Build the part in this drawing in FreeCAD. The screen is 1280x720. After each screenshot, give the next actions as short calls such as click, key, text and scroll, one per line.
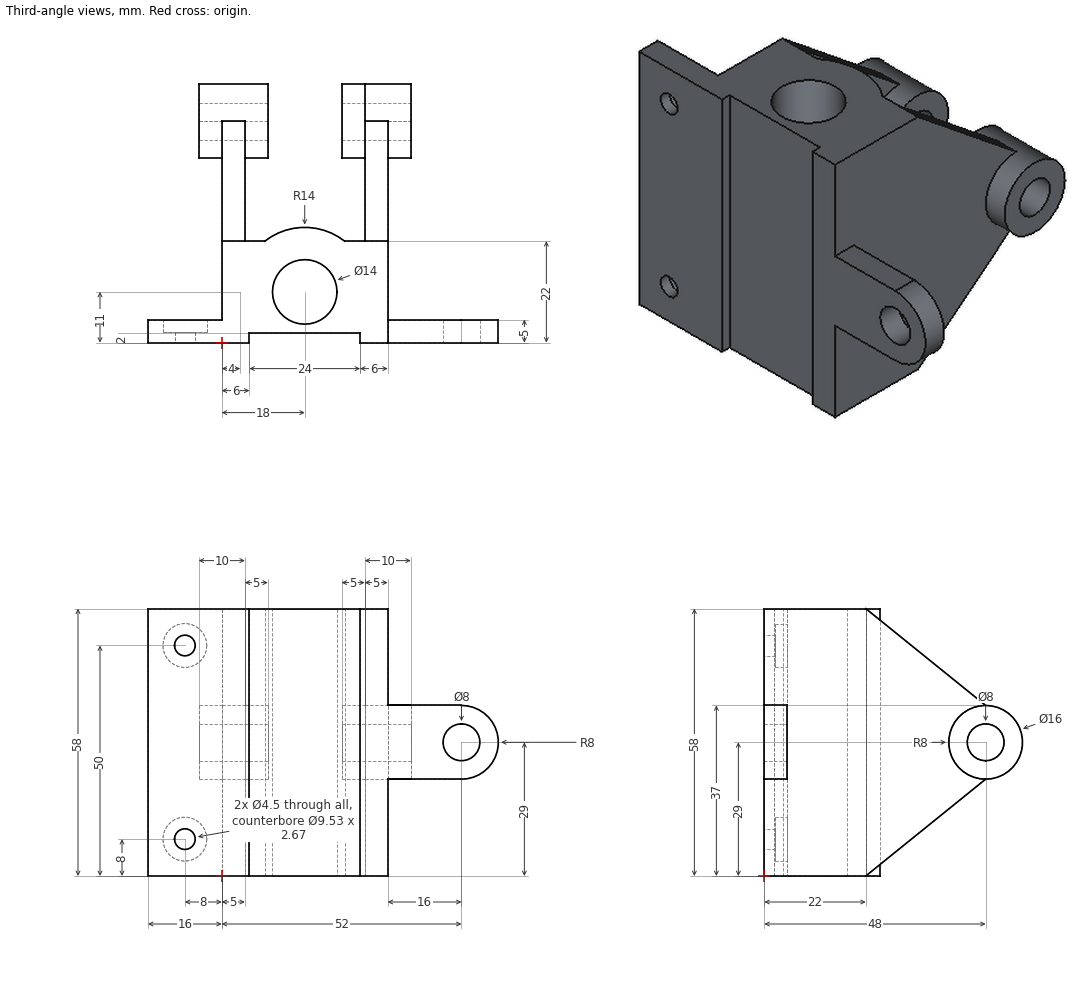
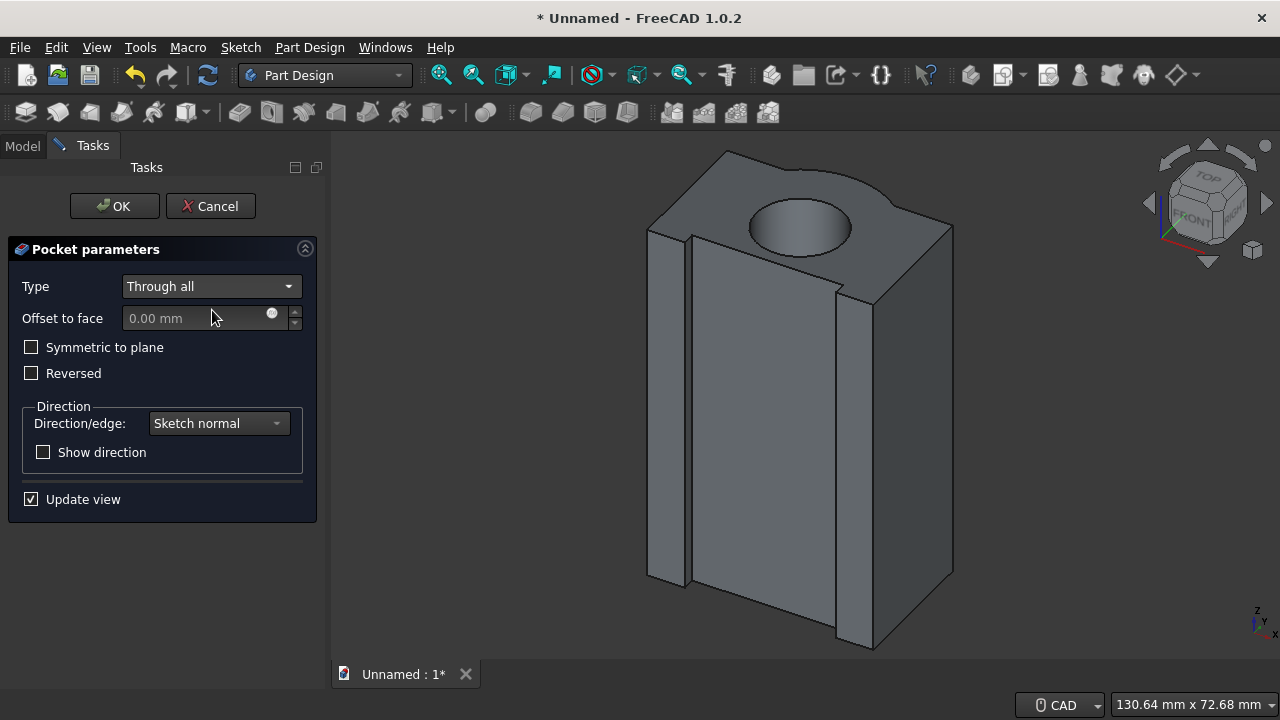
click(115, 206)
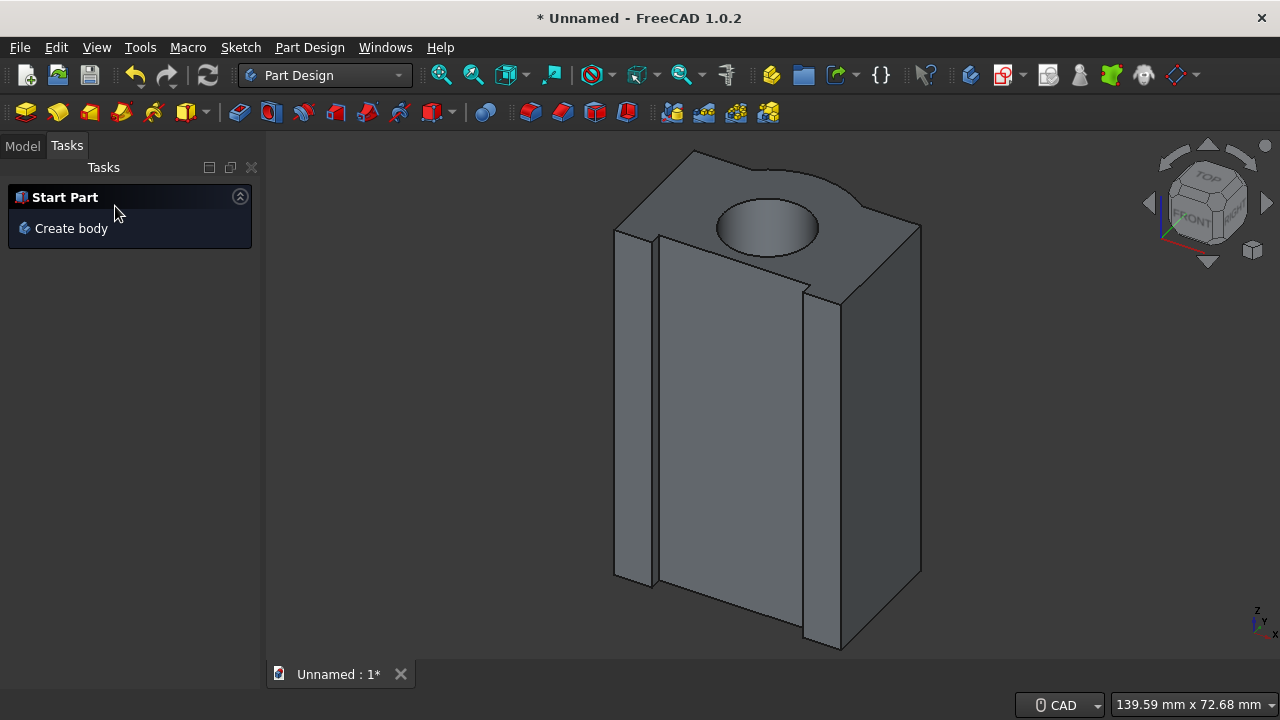
click(972, 76)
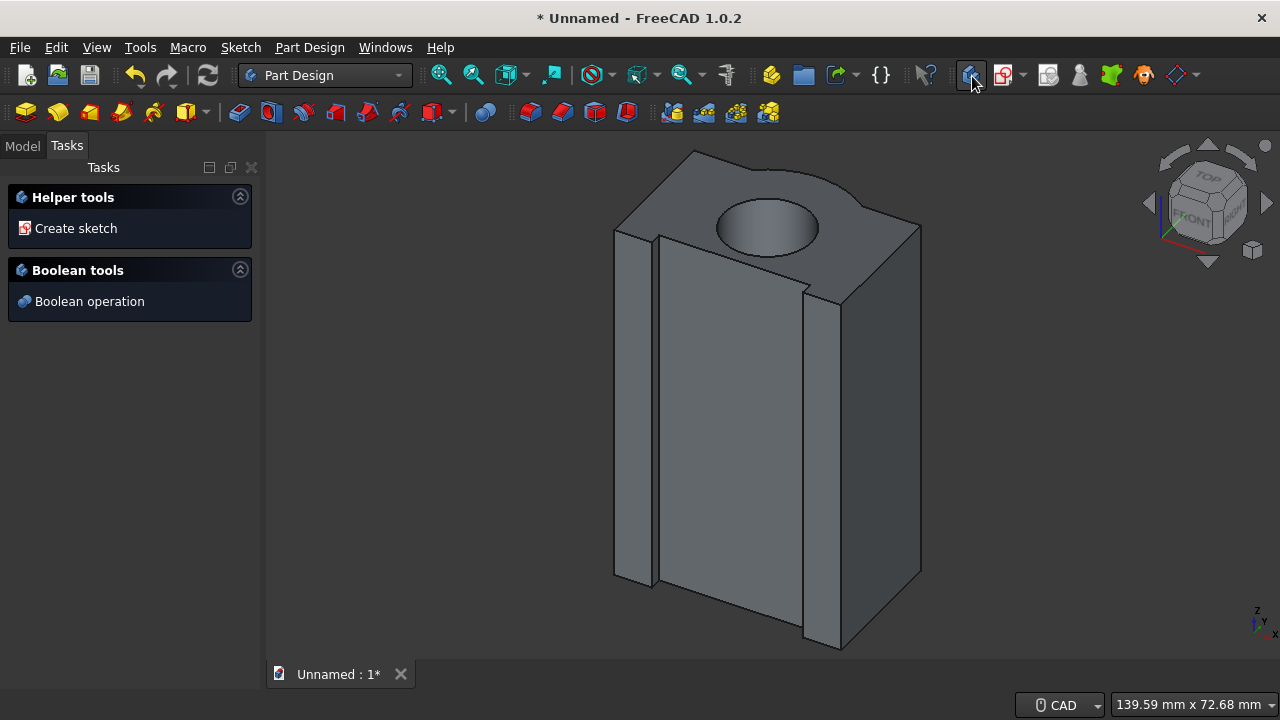
click(306, 619)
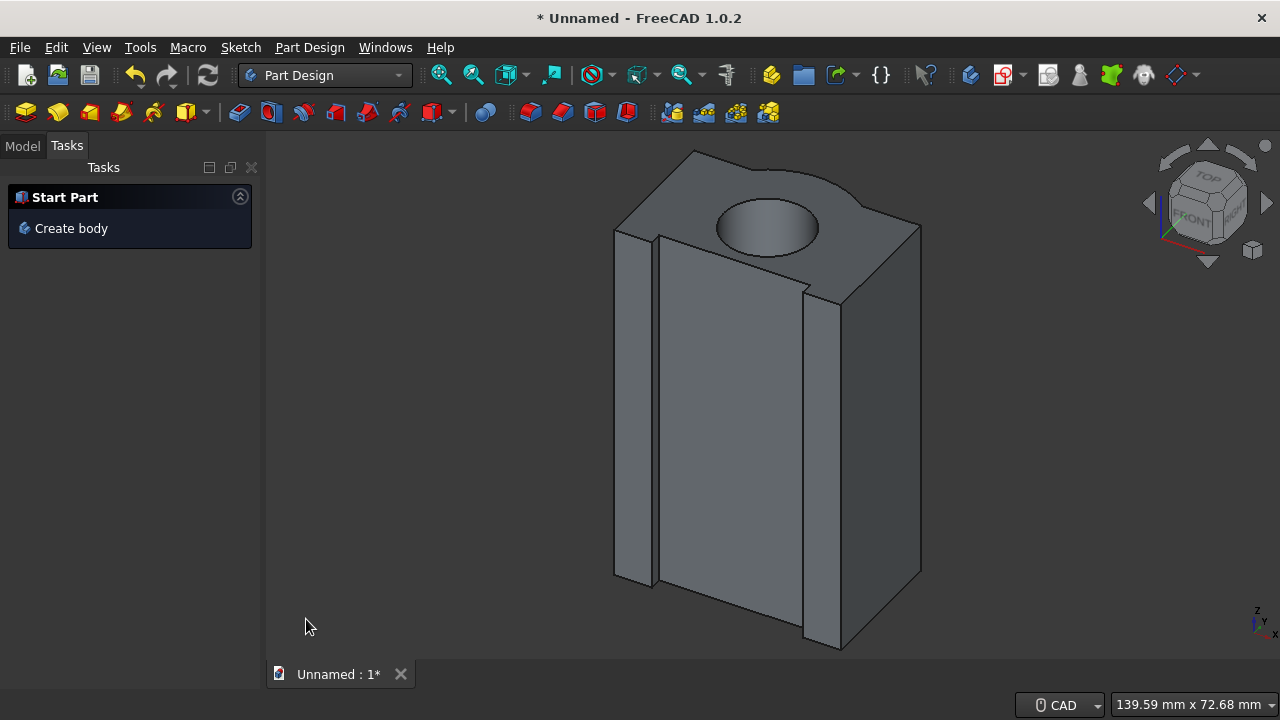
click(1004, 76)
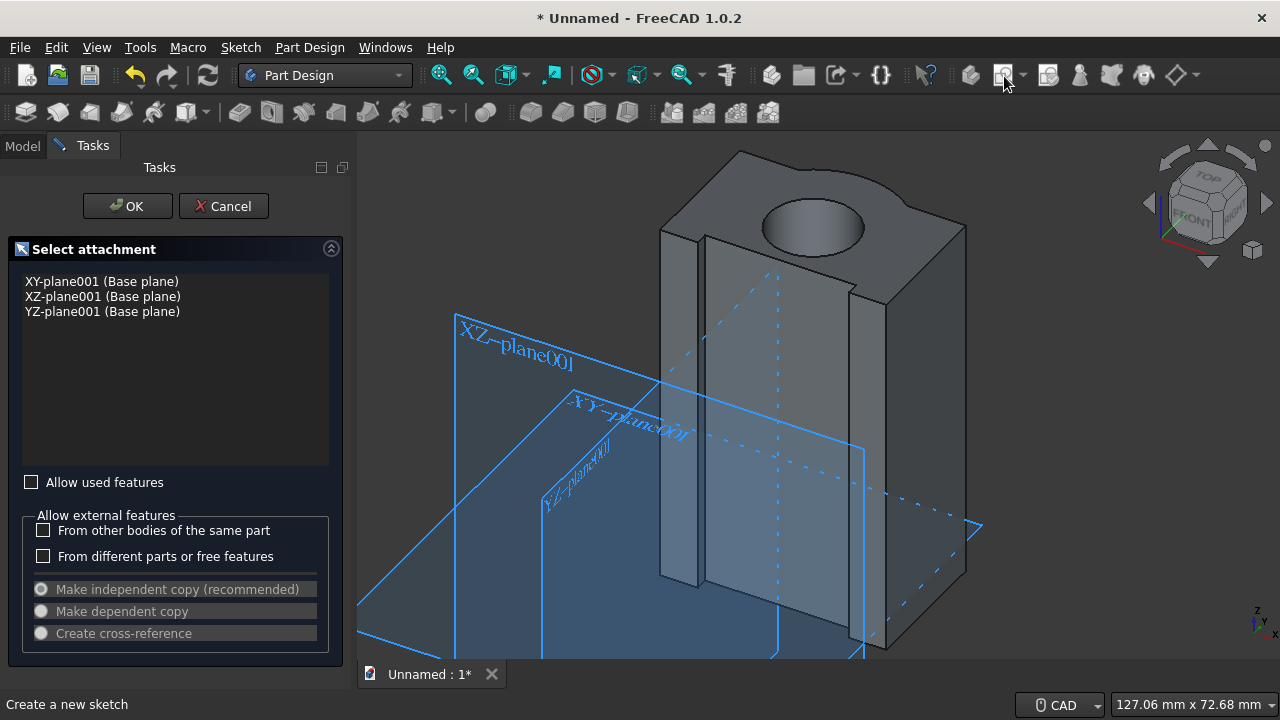
click(82, 312)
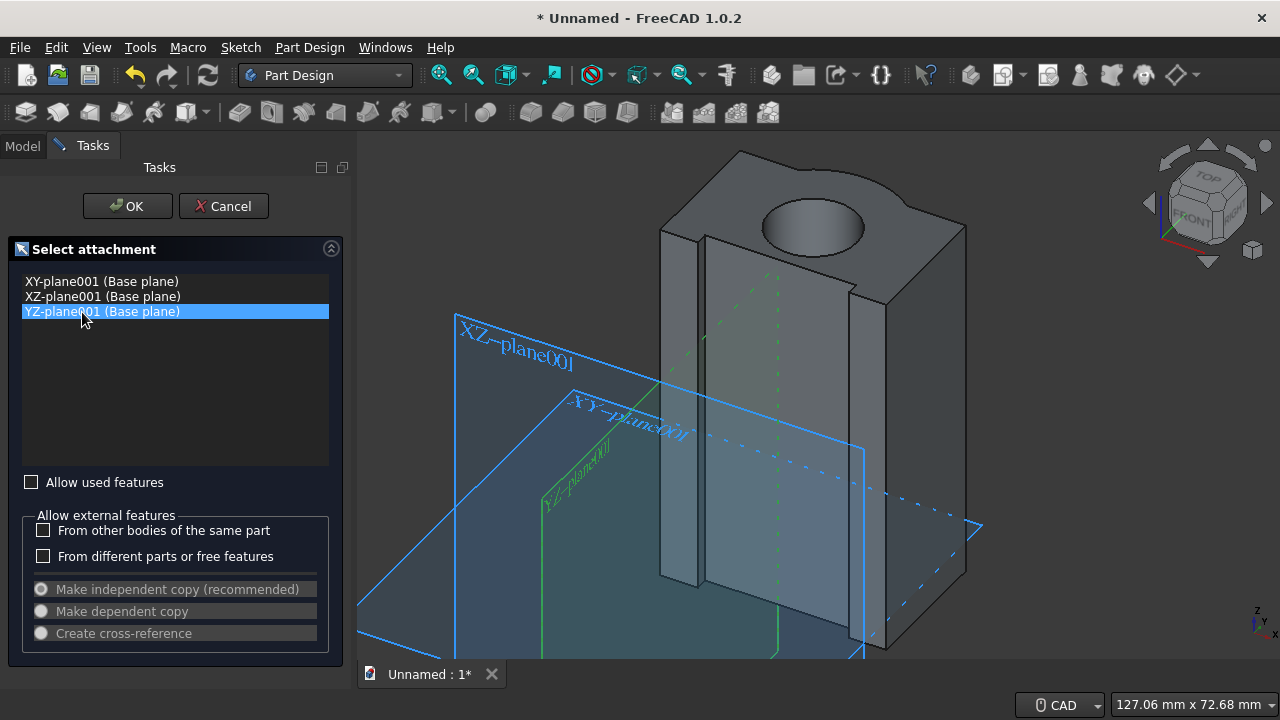
click(128, 206)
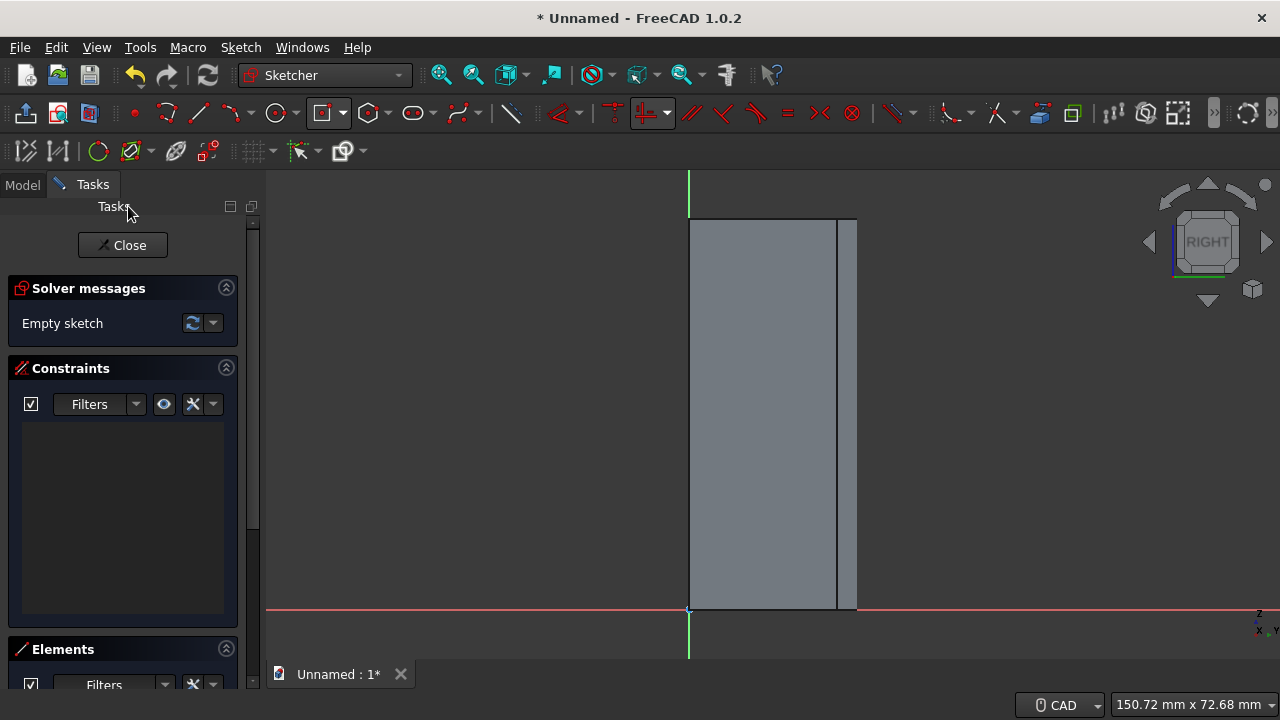
scroll(1115, 415, up, 5)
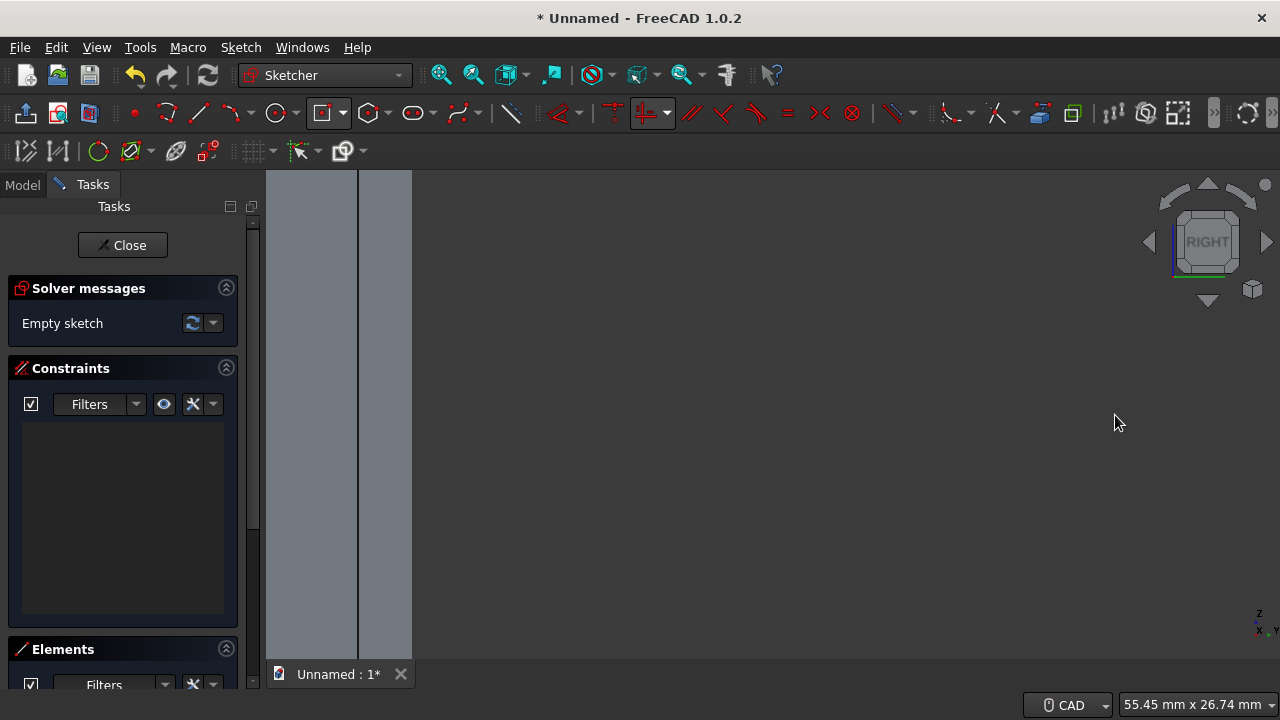
key(g)
key(c)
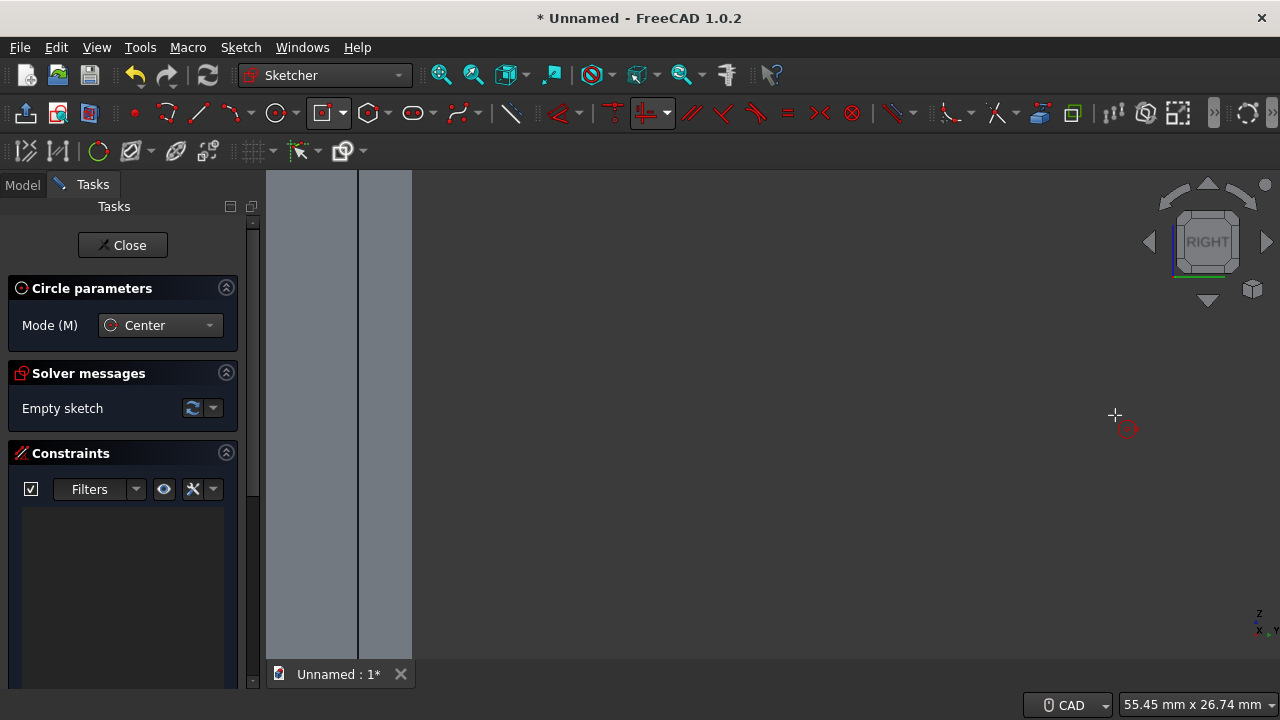
click(833, 413)
move(937, 309)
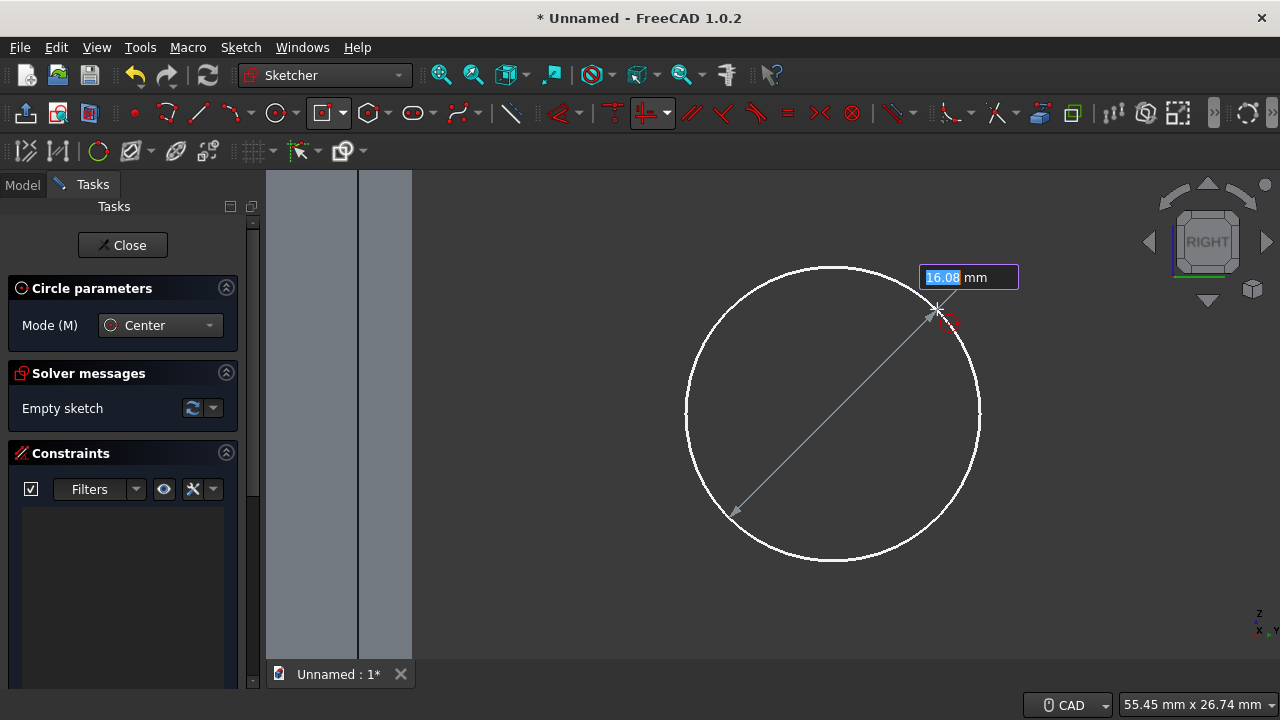
text(16)
key(Return)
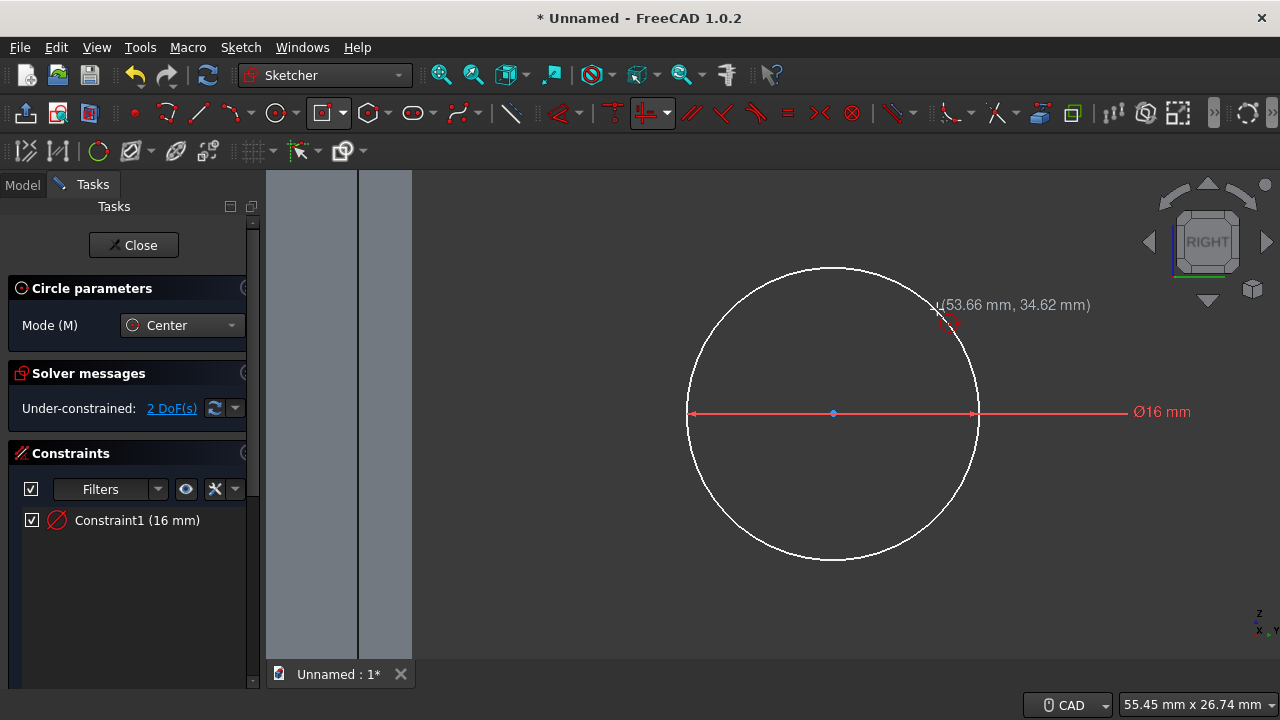
click(833, 414)
move(885, 361)